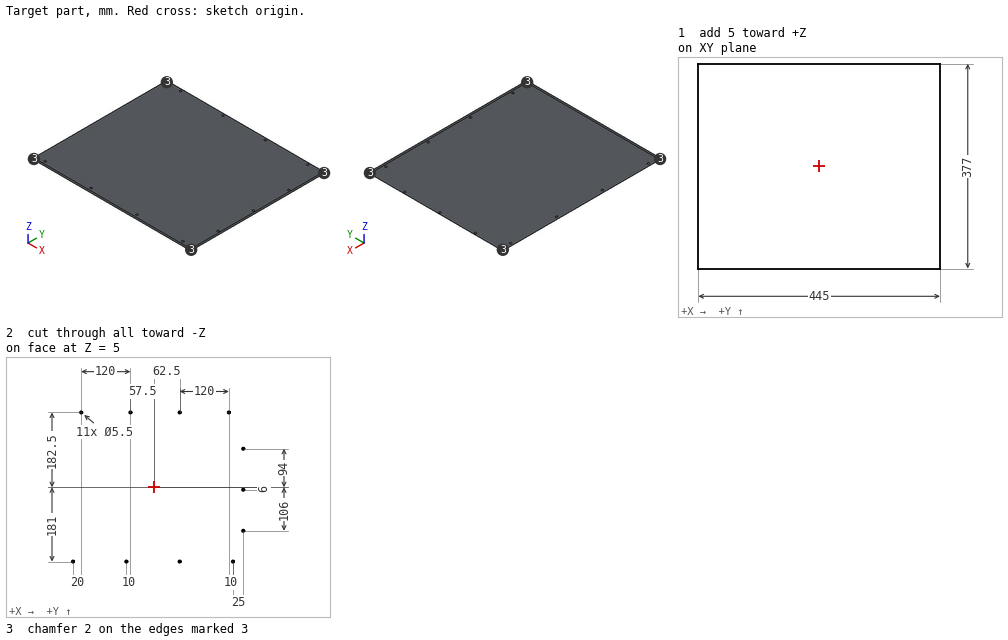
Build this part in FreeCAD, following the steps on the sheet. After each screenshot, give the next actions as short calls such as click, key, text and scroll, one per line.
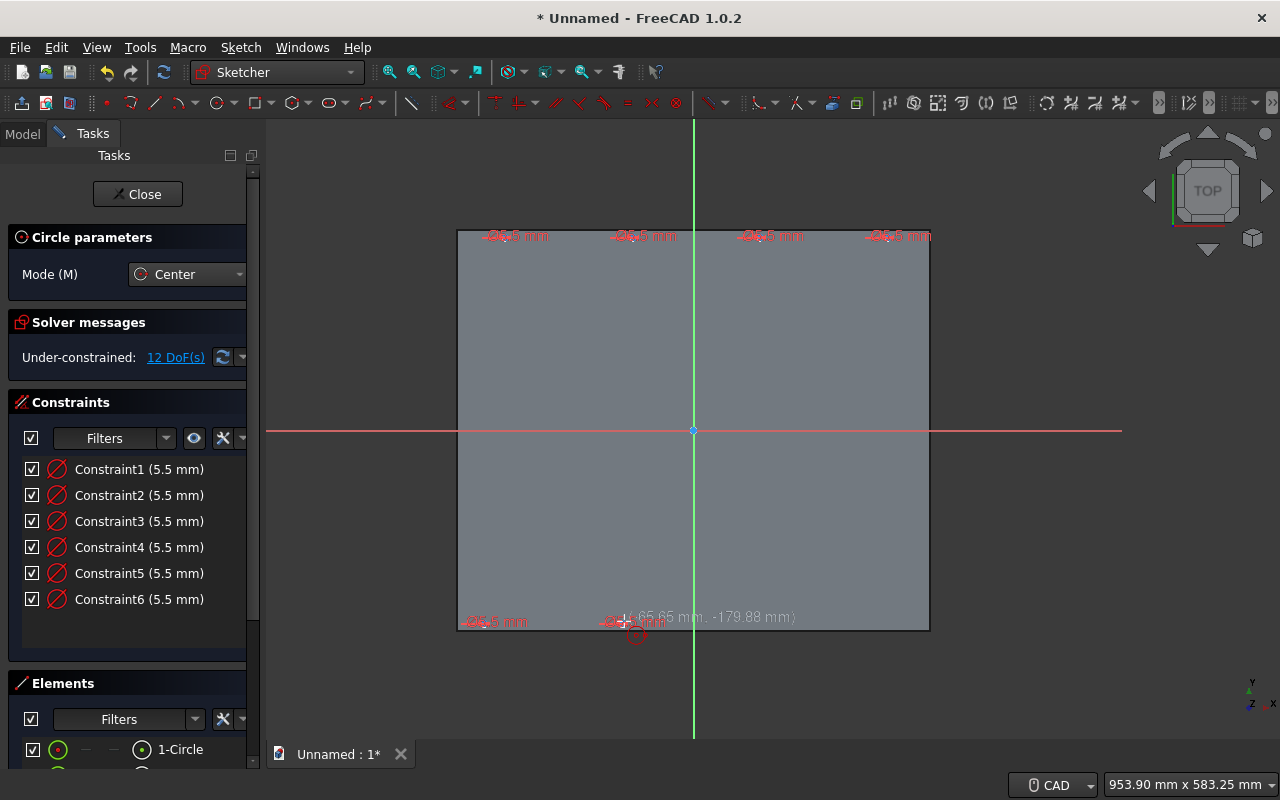
scroll(760, 623, up, 11)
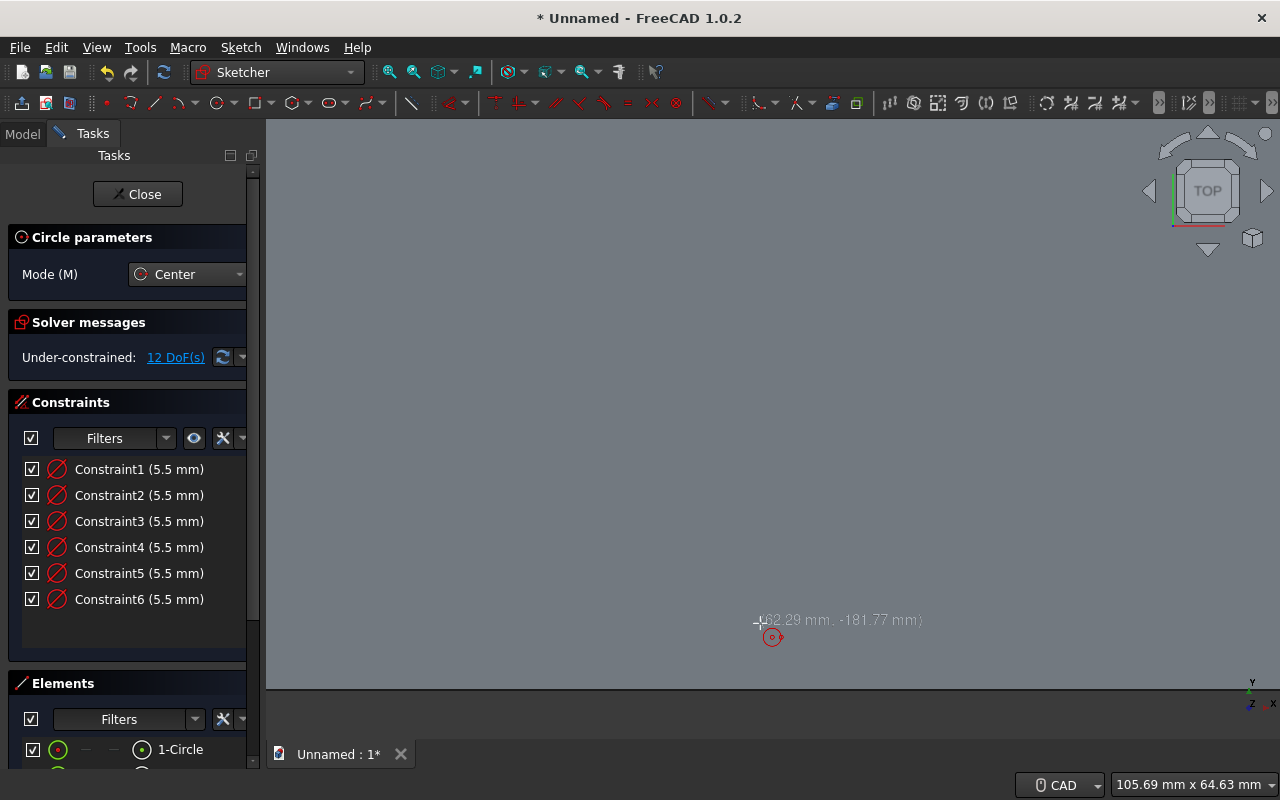
scroll(761, 623, down, 11)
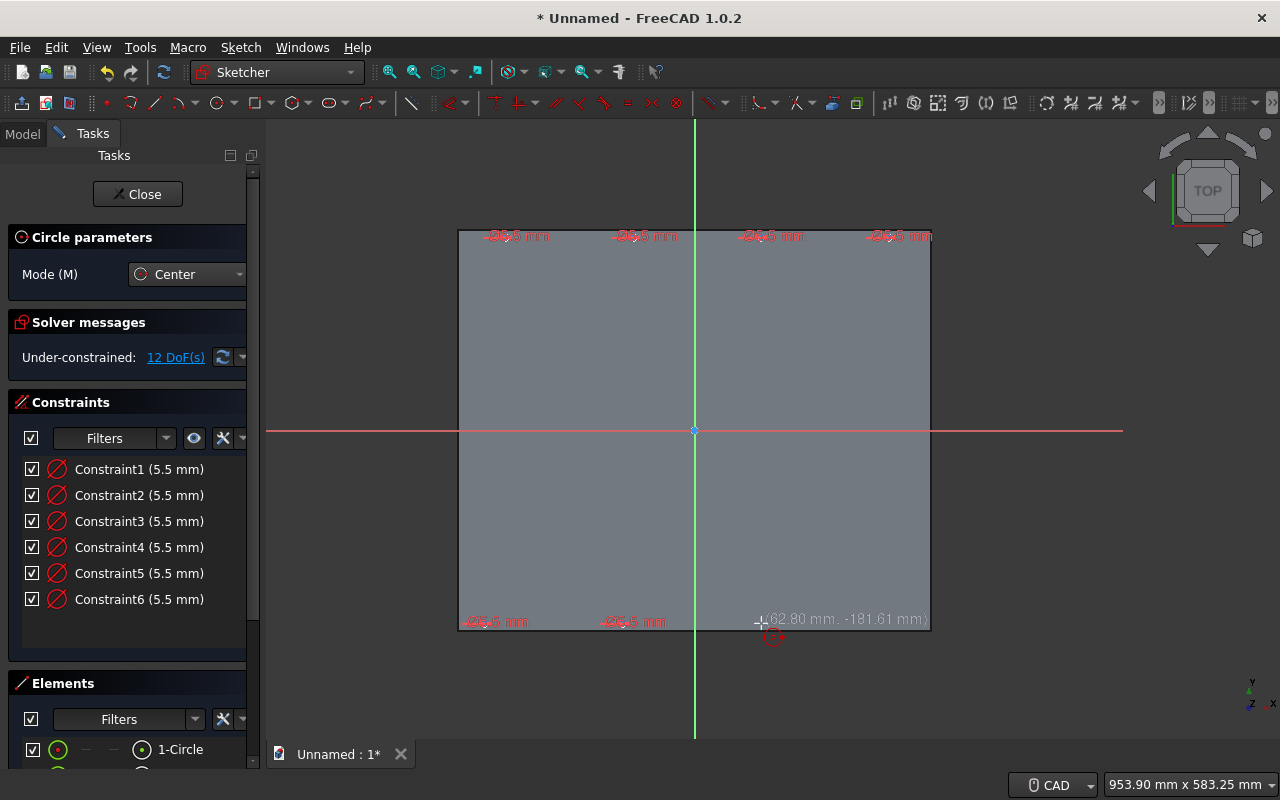
click(761, 623)
move(763, 621)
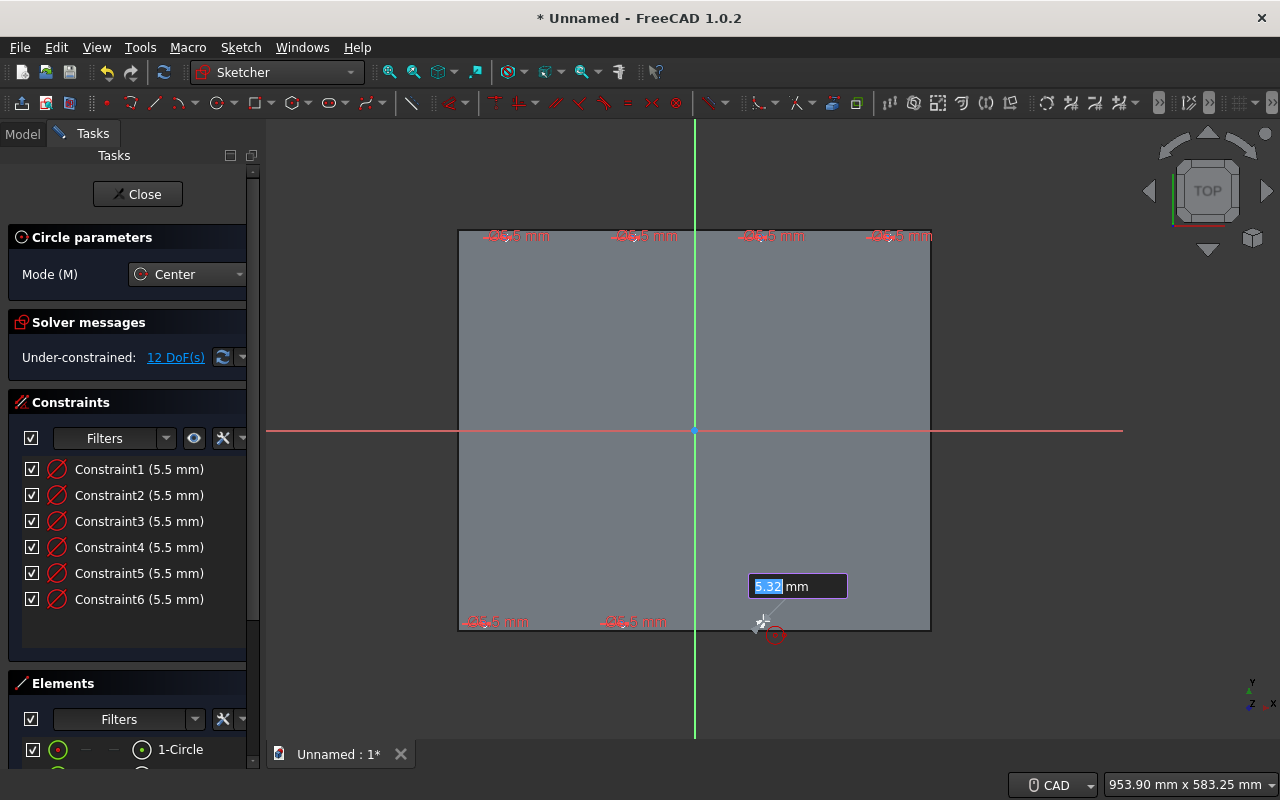
text(5.5)
key(Return)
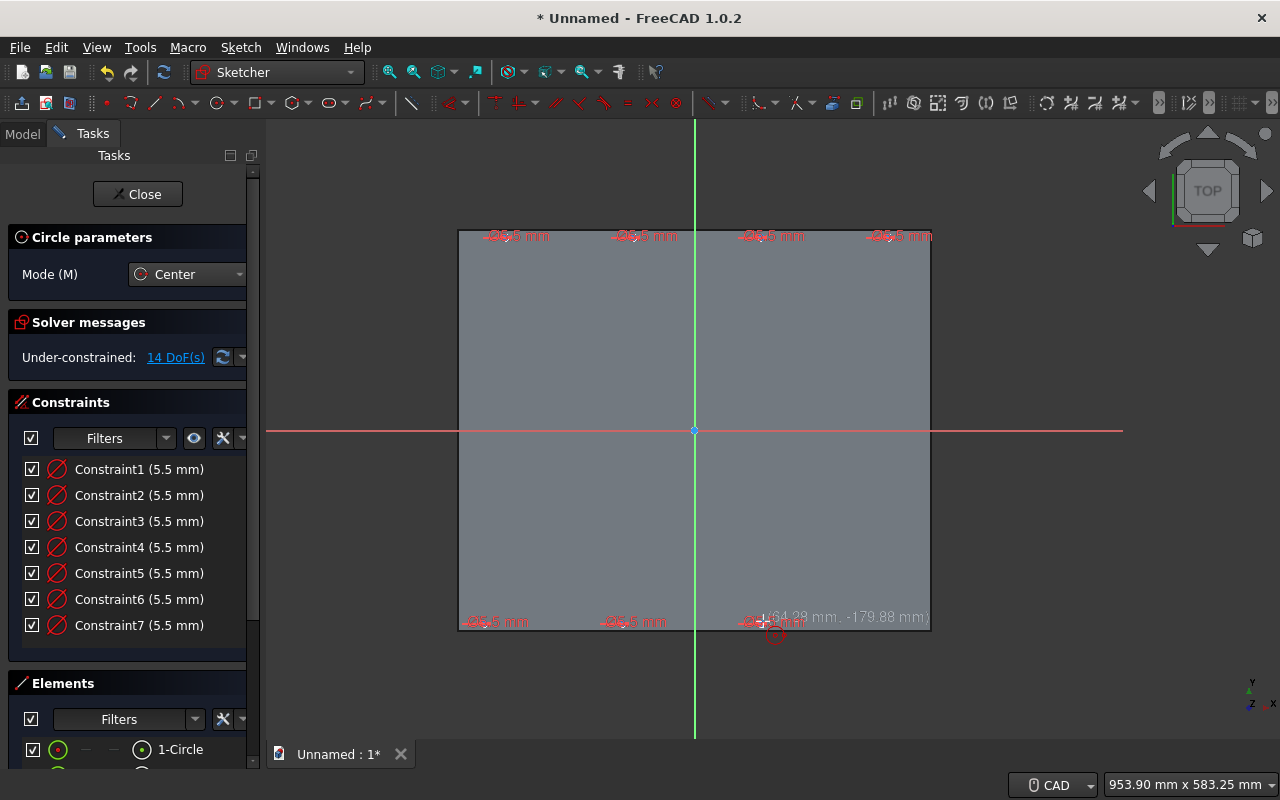
scroll(899, 623, up, 11)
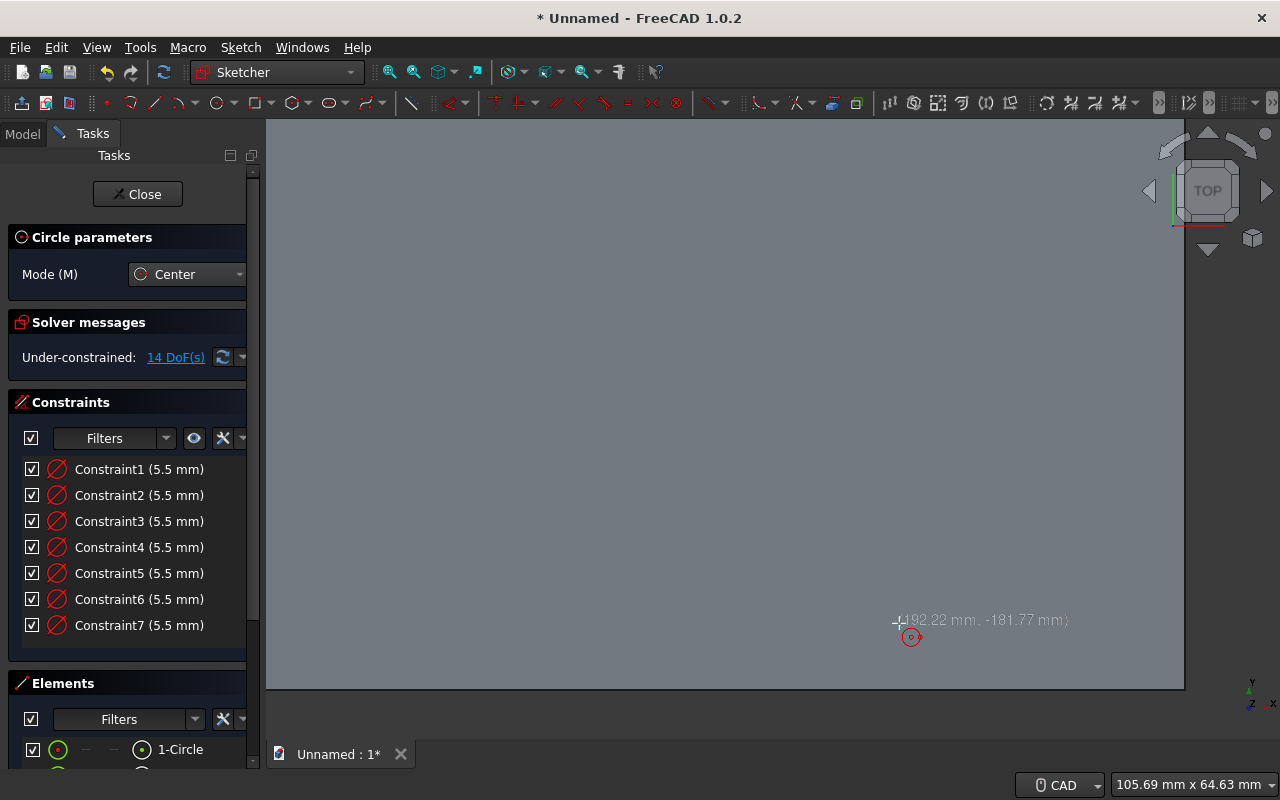
scroll(899, 623, down, 11)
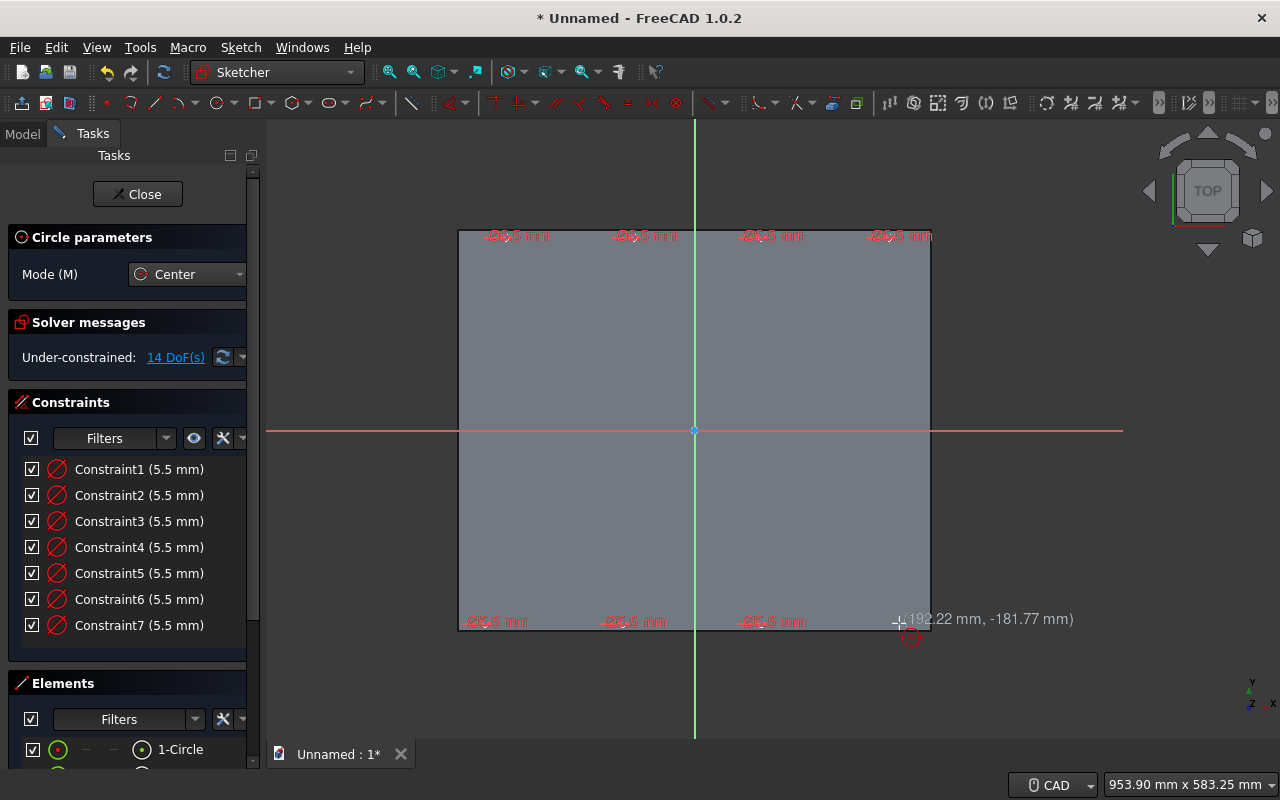
click(899, 623)
move(901, 621)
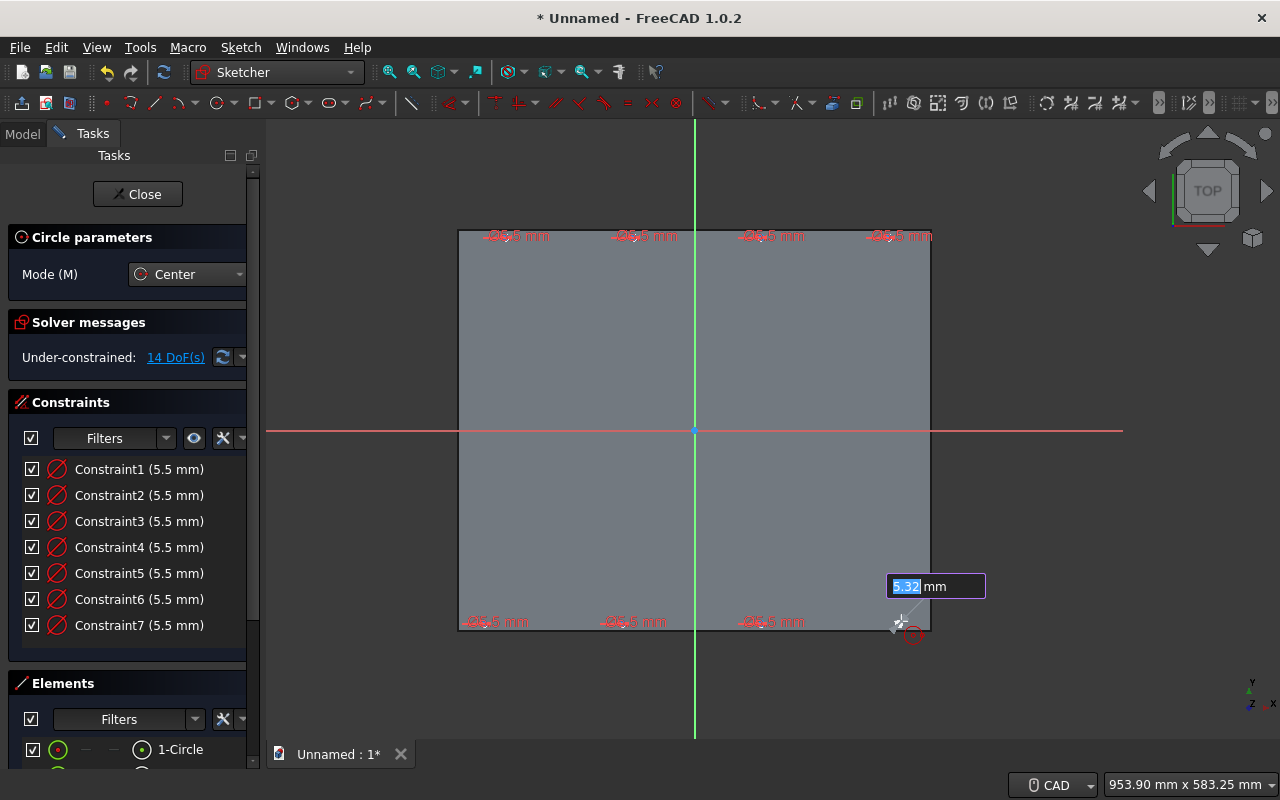
text(5.5)
key(Return)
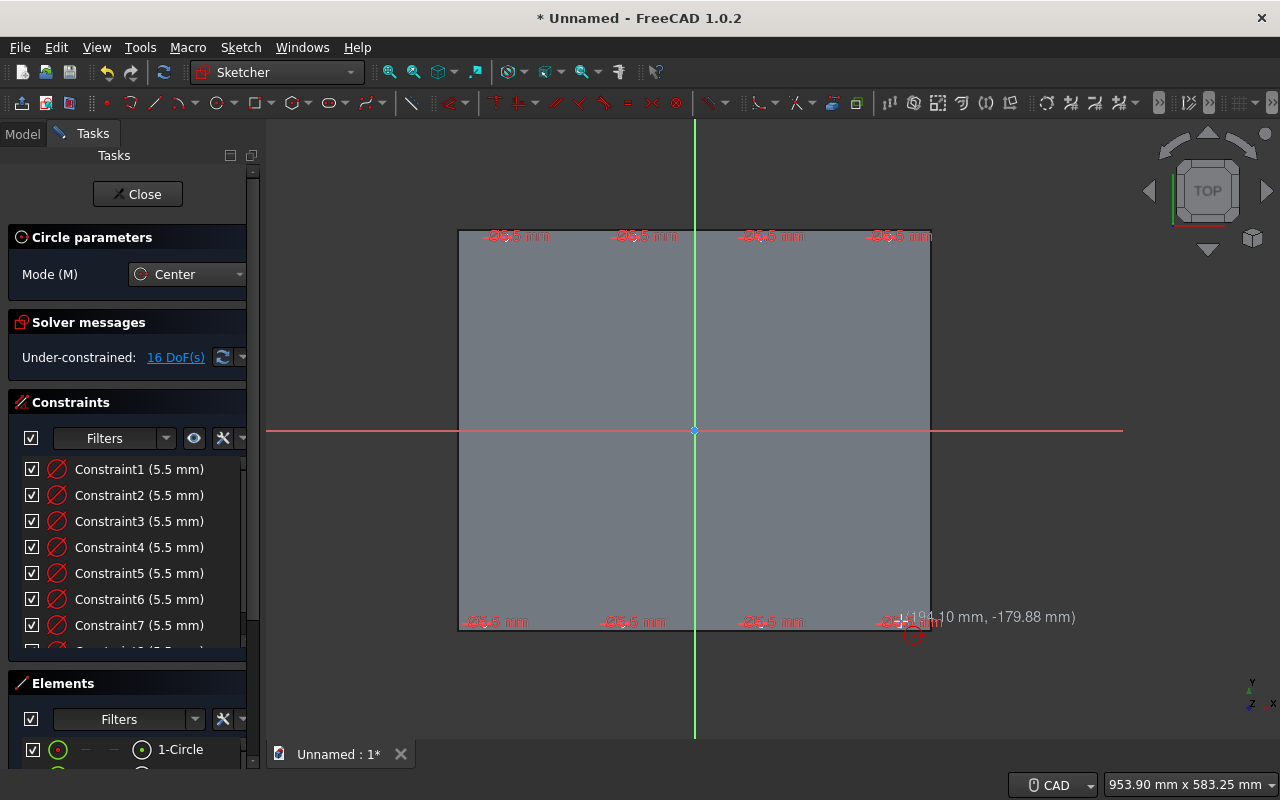
scroll(926, 543, up, 11)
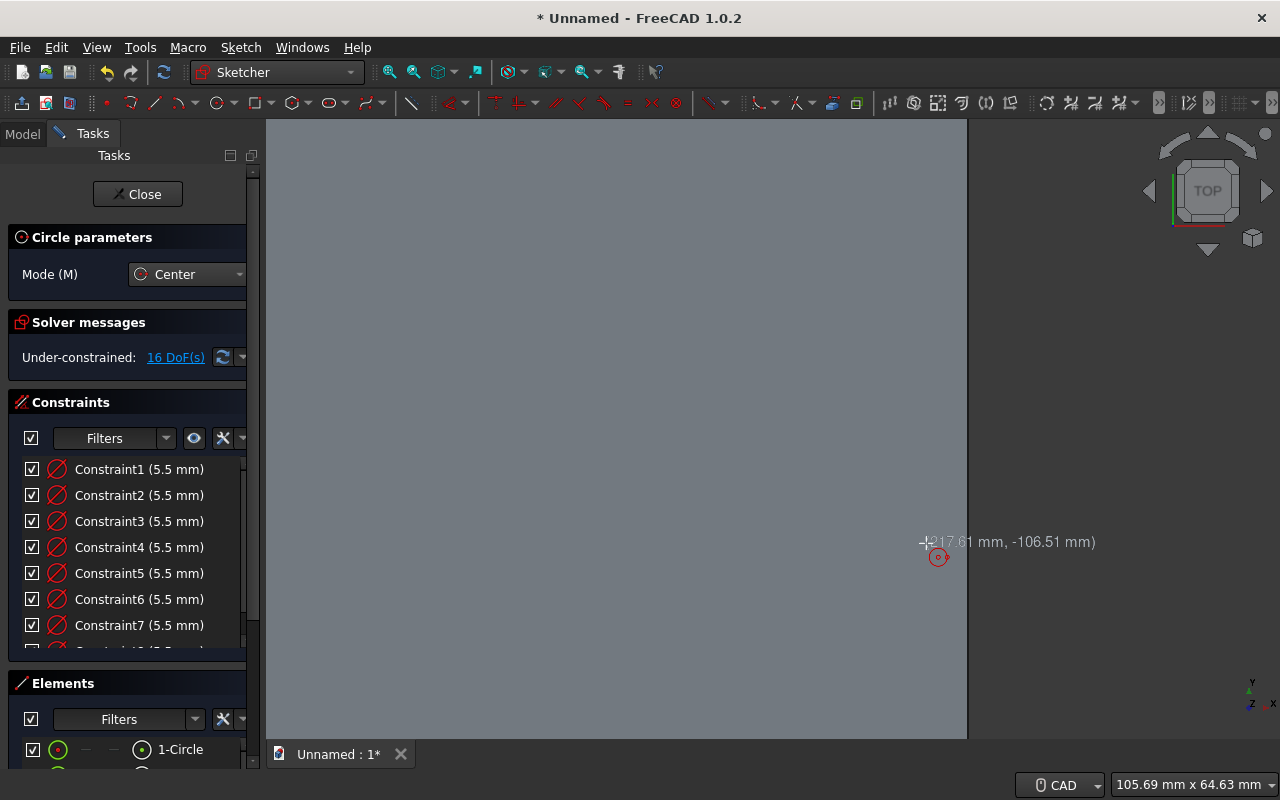
scroll(926, 543, down, 11)